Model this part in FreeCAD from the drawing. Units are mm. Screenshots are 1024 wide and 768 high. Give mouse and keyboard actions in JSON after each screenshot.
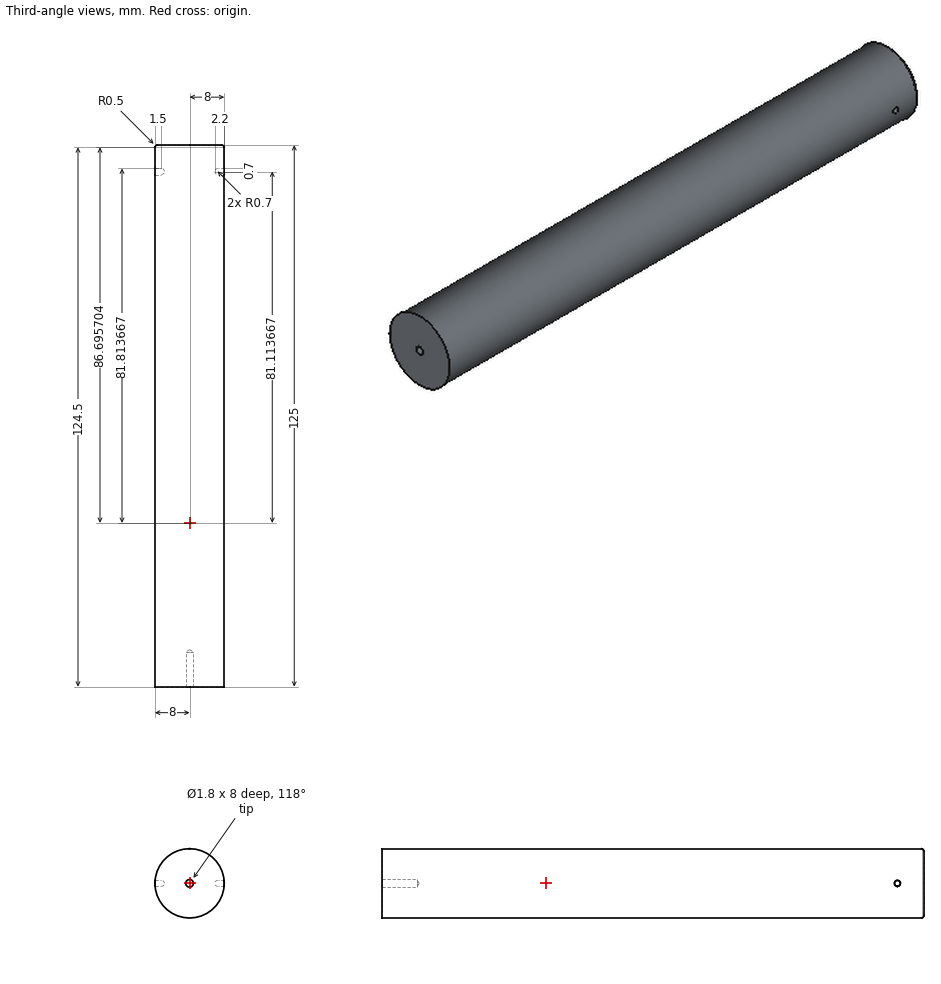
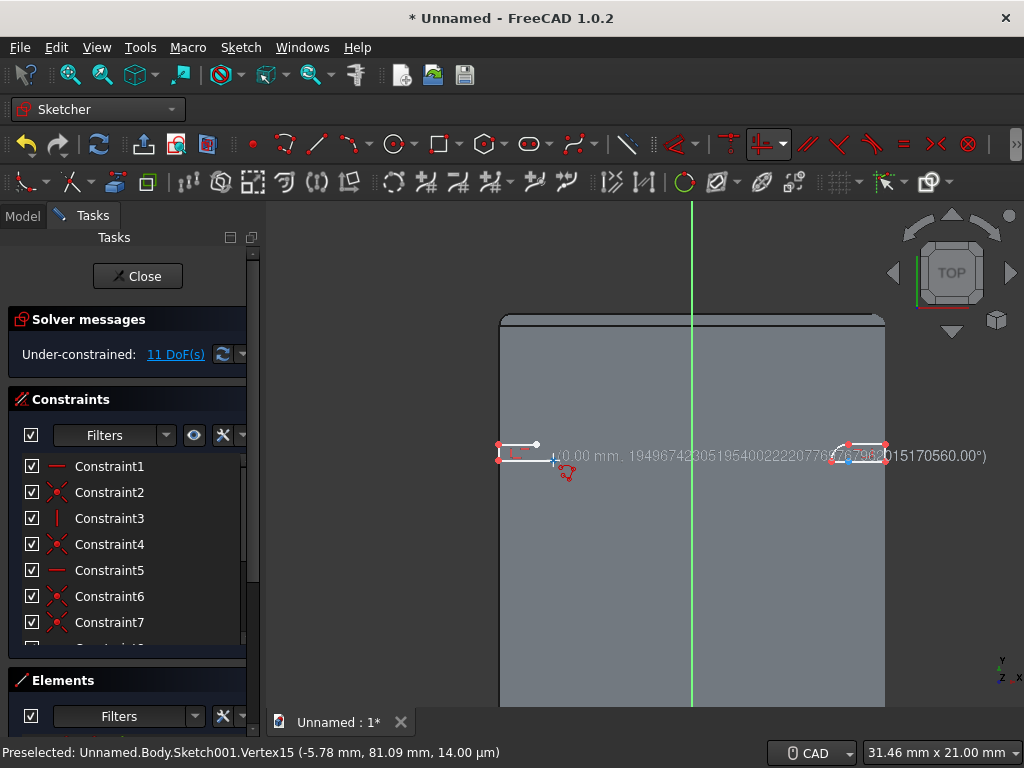
{"action": "key", "text": "g 3 a"}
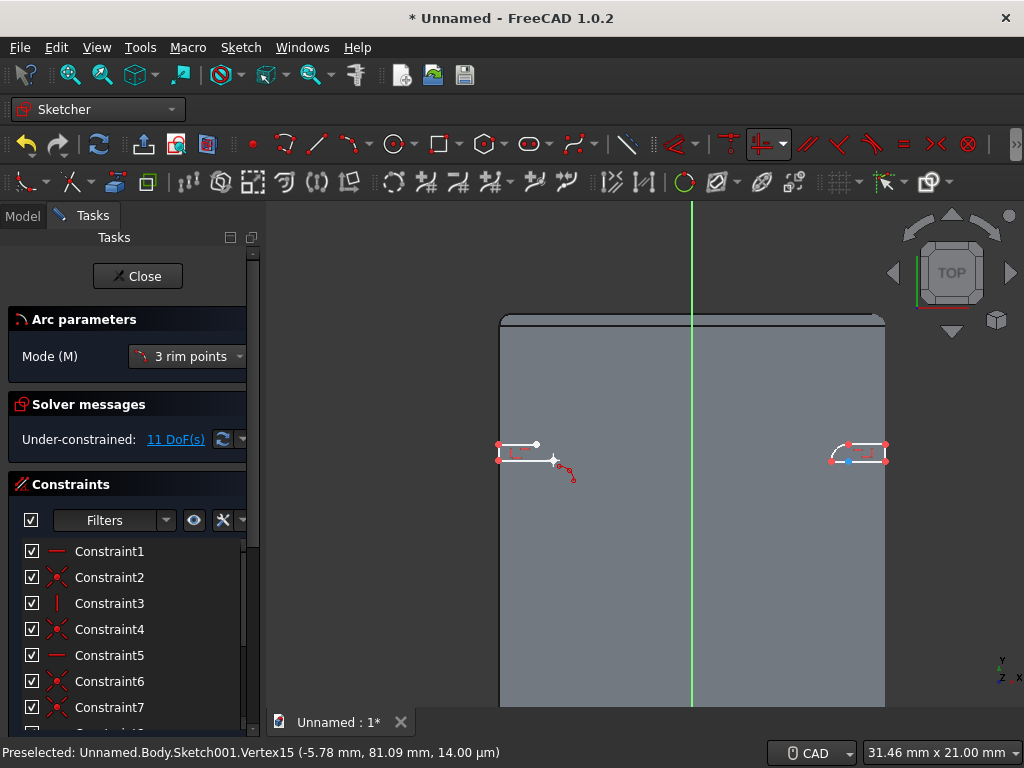
{"action": "left_click", "coordinate": [553, 461]}
{"action": "left_click", "coordinate": [536, 445]}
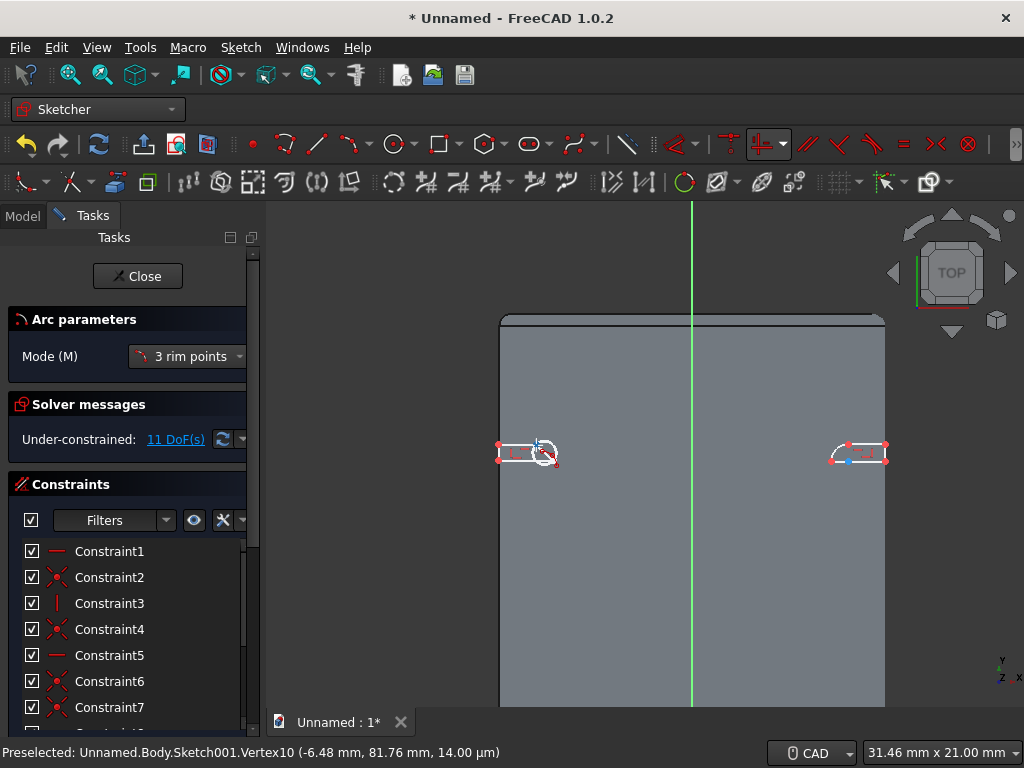
{"action": "scroll", "coordinate": [548, 448], "scroll_direction": "up", "scroll_amount": 6}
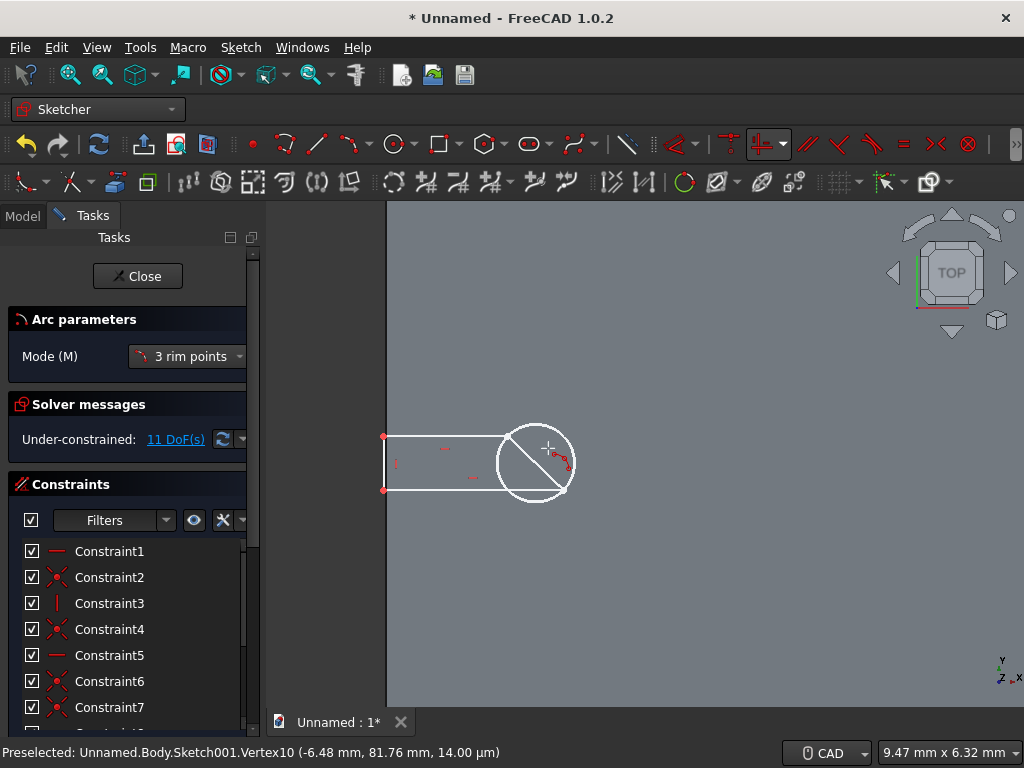
{"action": "left_click", "coordinate": [546, 448]}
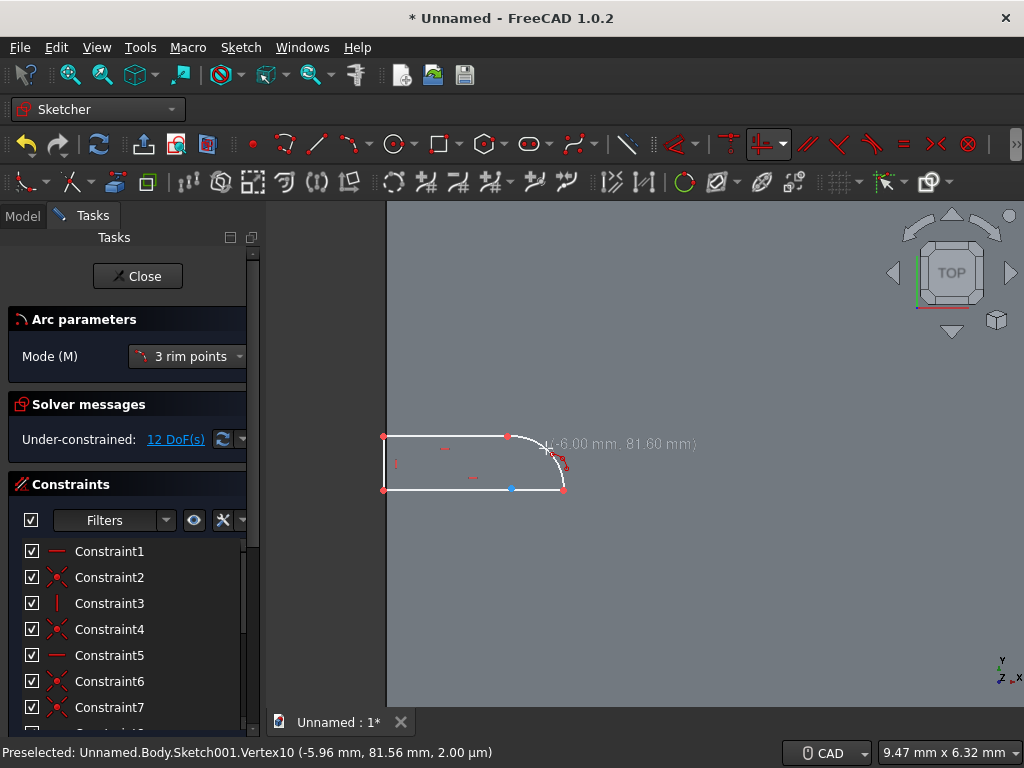
{"action": "key", "text": "g l"}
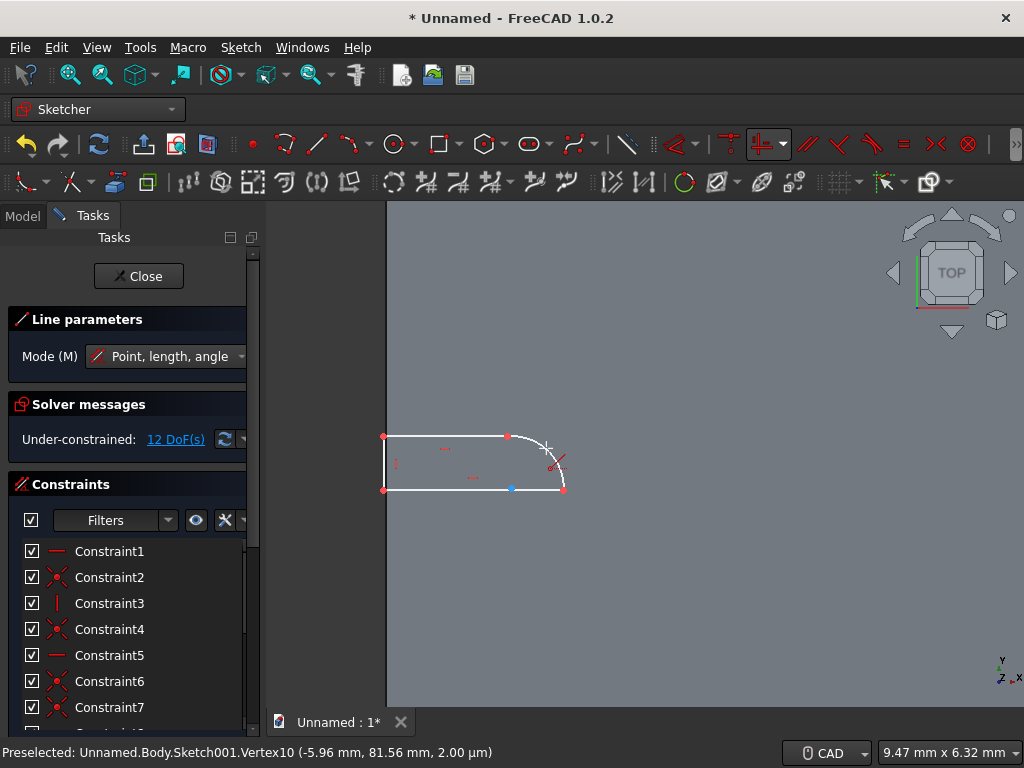
{"action": "scroll", "coordinate": [528, 453], "scroll_direction": "down", "scroll_amount": 8}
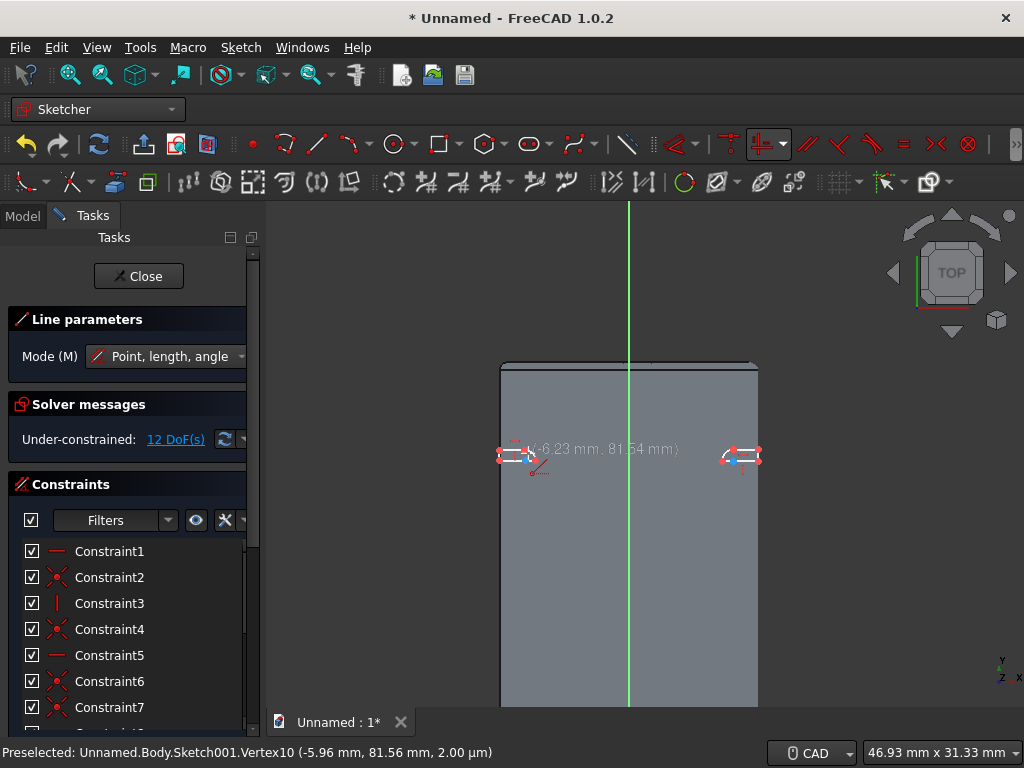
{"action": "left_click", "coordinate": [474, 460]}
{"action": "left_click", "coordinate": [396, 460]}
{"action": "key", "text": "Escape"}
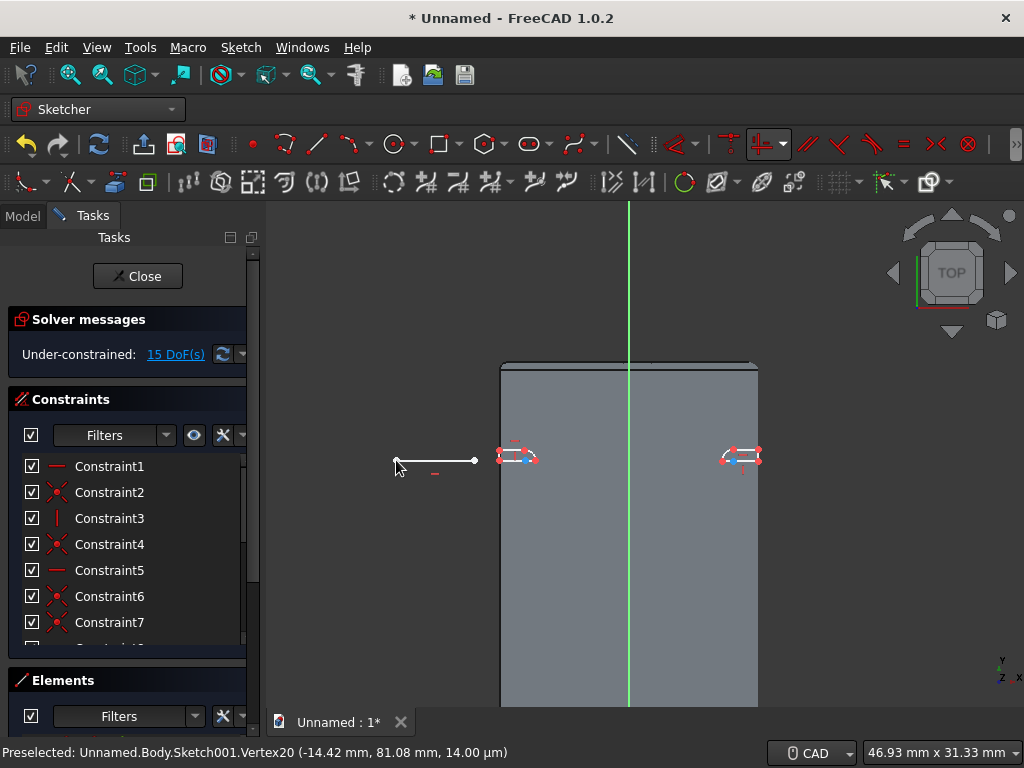
{"action": "left_click", "coordinate": [451, 461]}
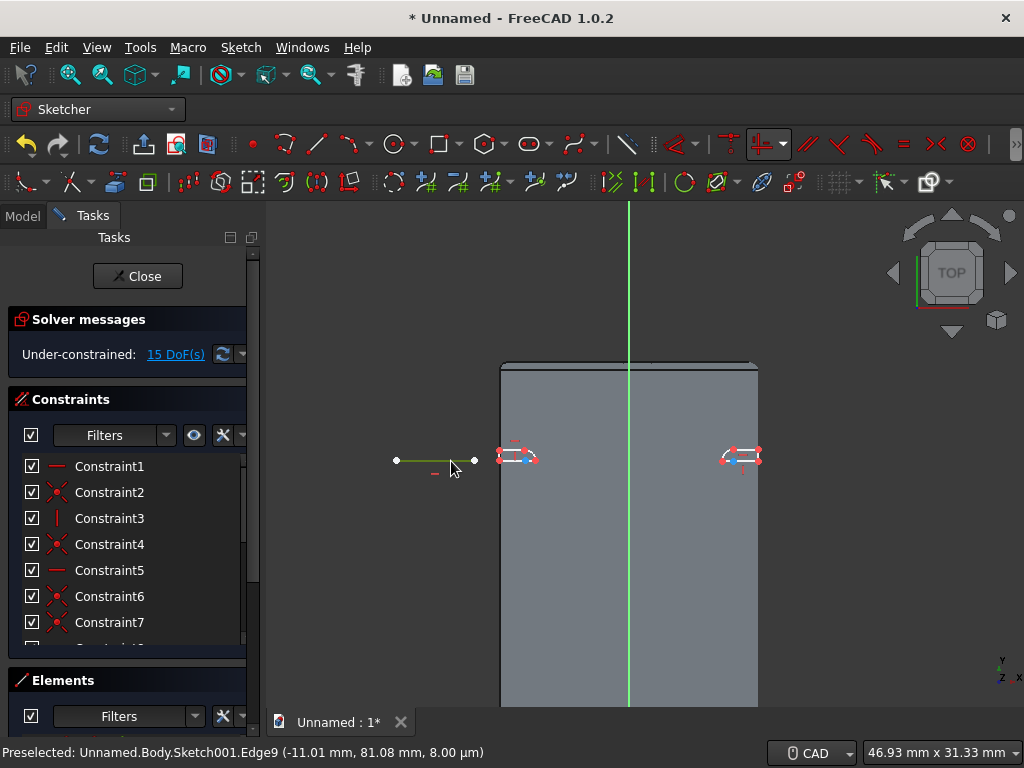
{"action": "left_click", "coordinate": [628, 144]}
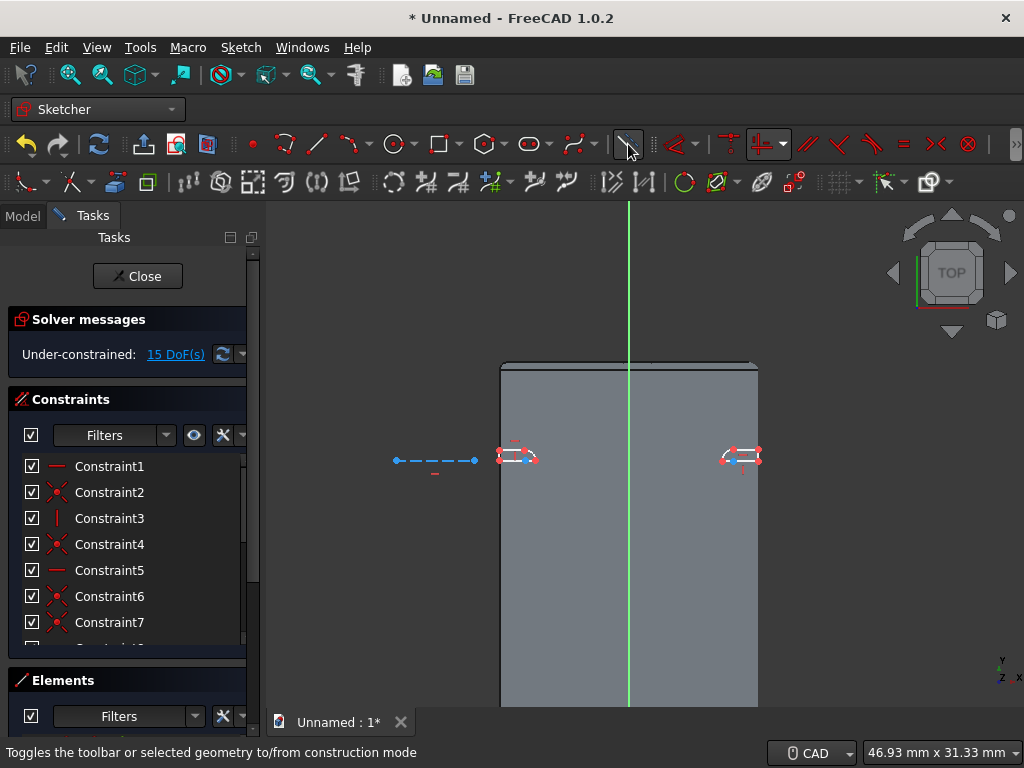
{"action": "scroll", "coordinate": [748, 450], "scroll_direction": "up", "scroll_amount": 2}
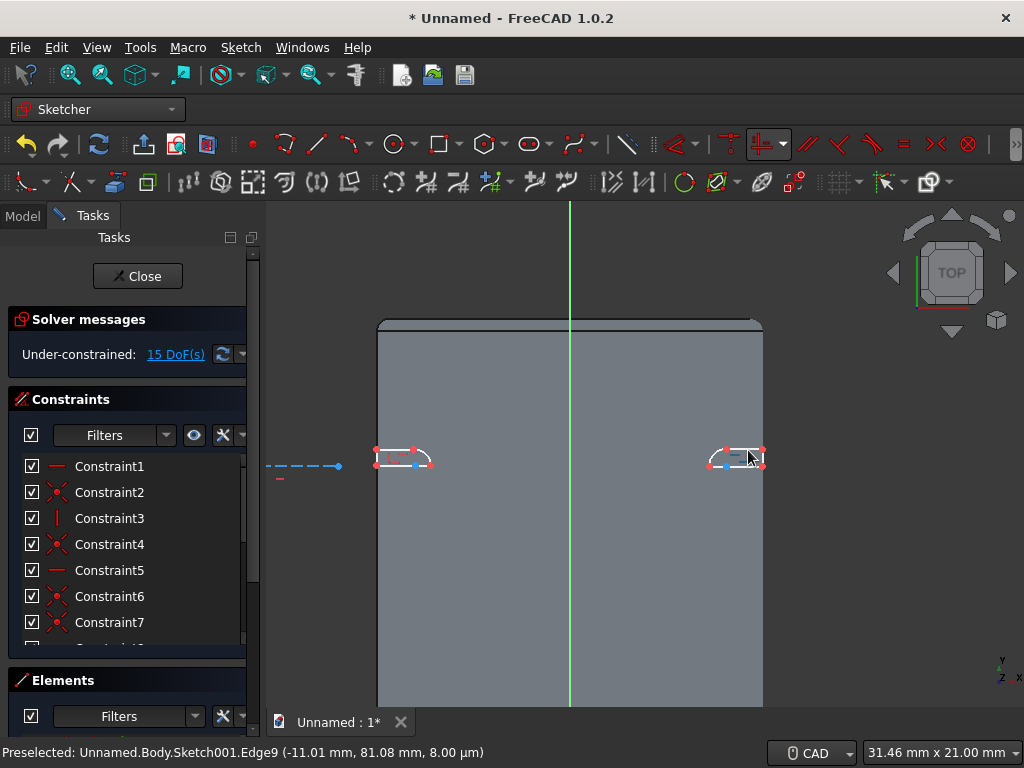
{"action": "left_click", "coordinate": [748, 449]}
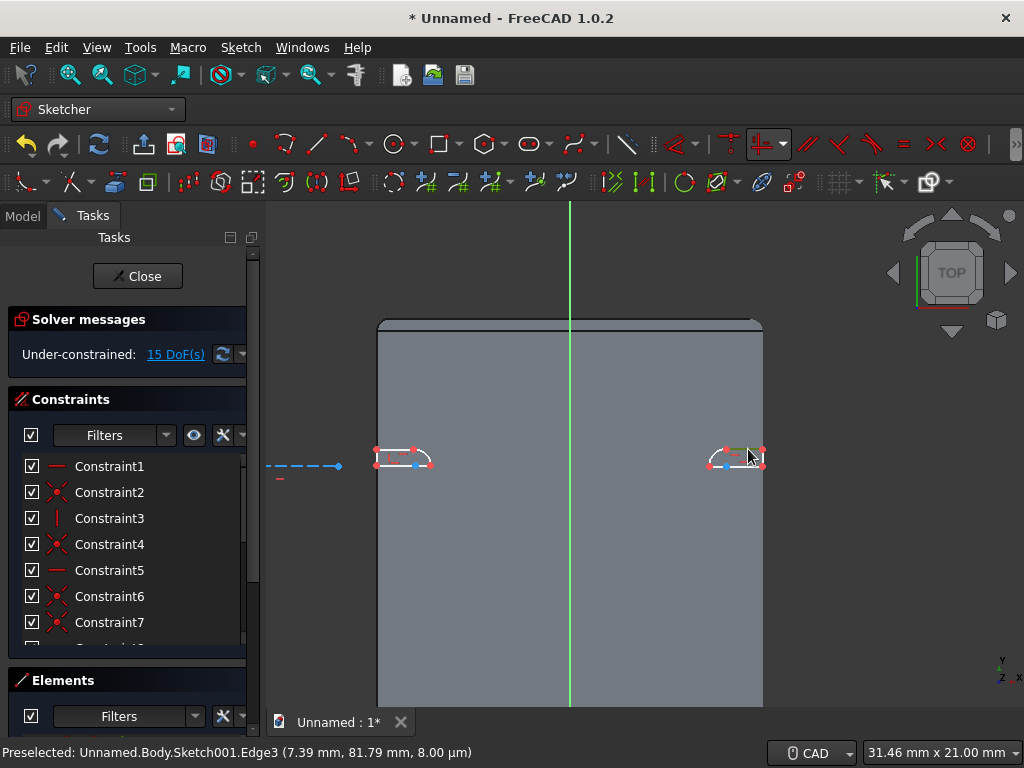
{"action": "left_click", "coordinate": [714, 454]}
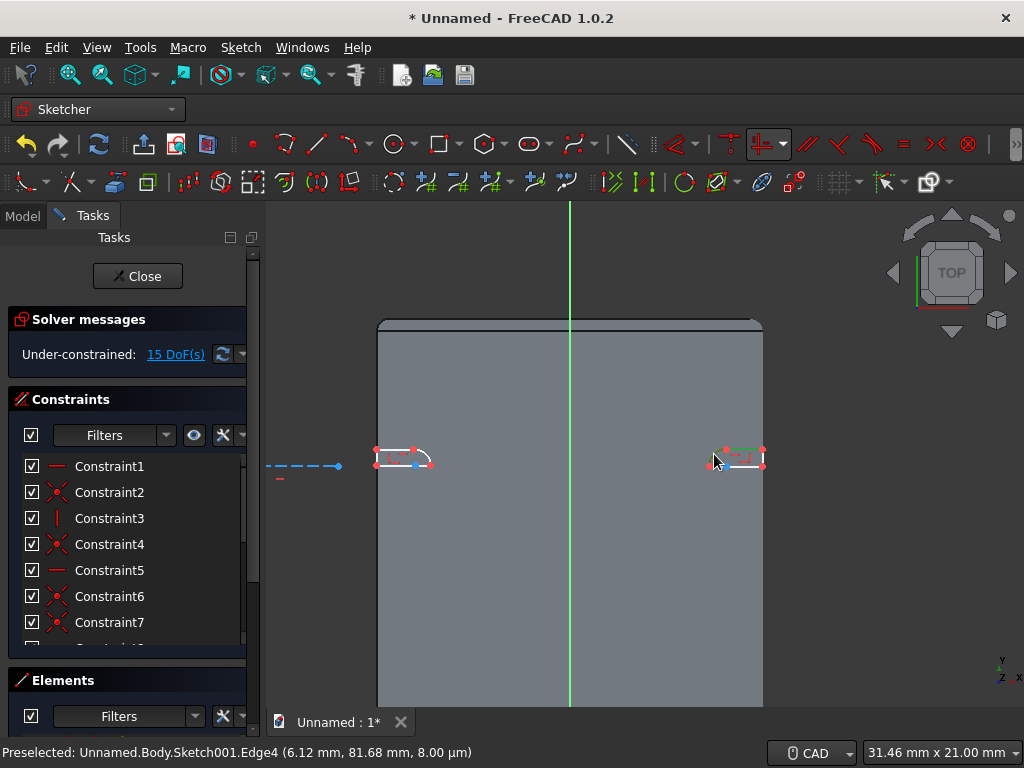
{"action": "key", "text": "t"}